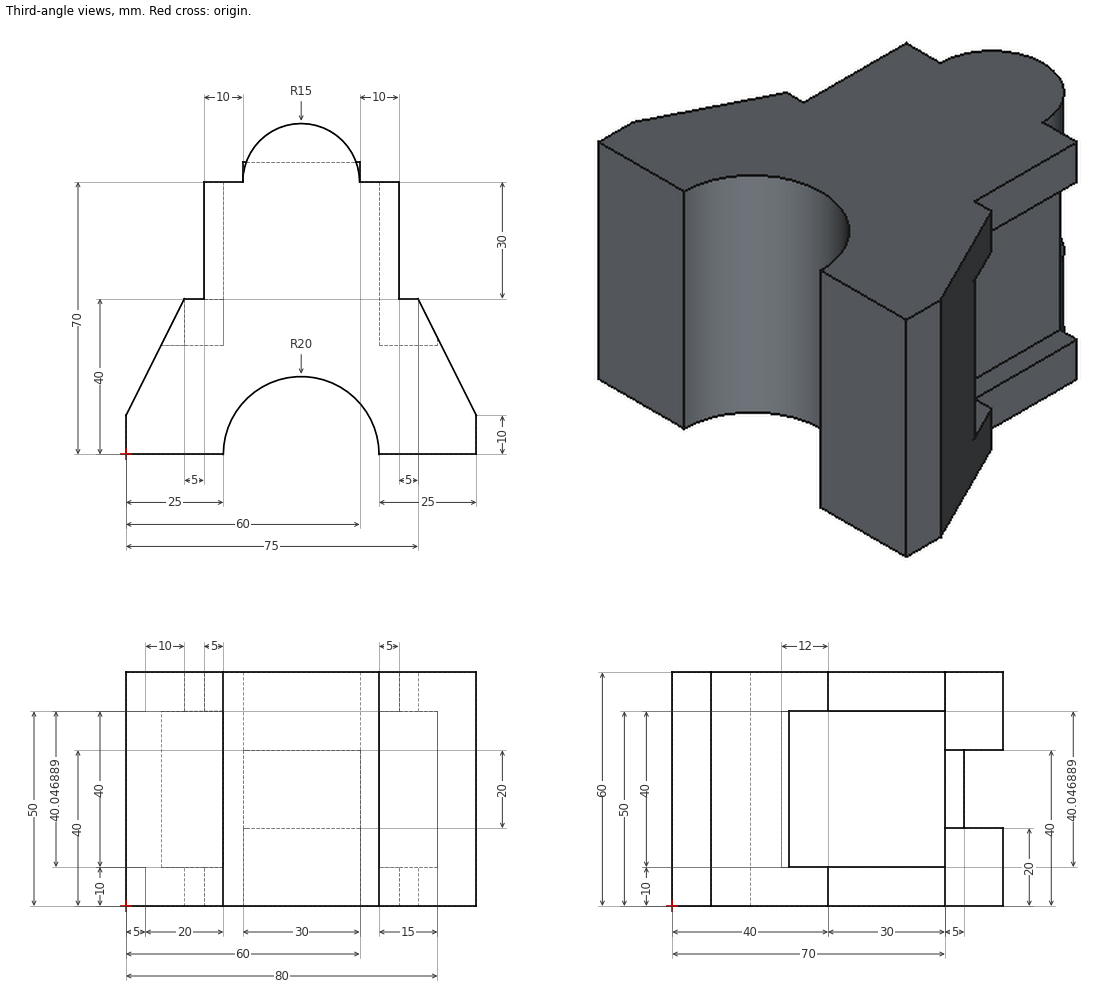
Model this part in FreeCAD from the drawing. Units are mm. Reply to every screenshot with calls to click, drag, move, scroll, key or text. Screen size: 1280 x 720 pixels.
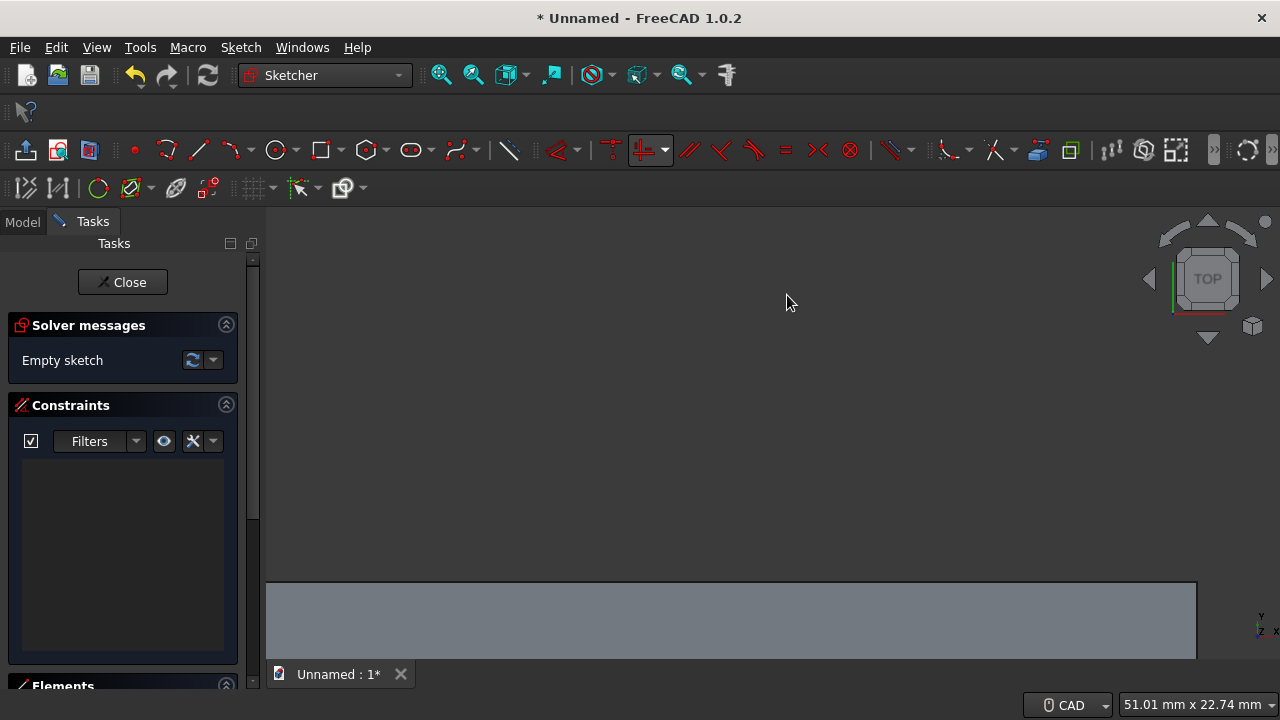
key(g)
key(l)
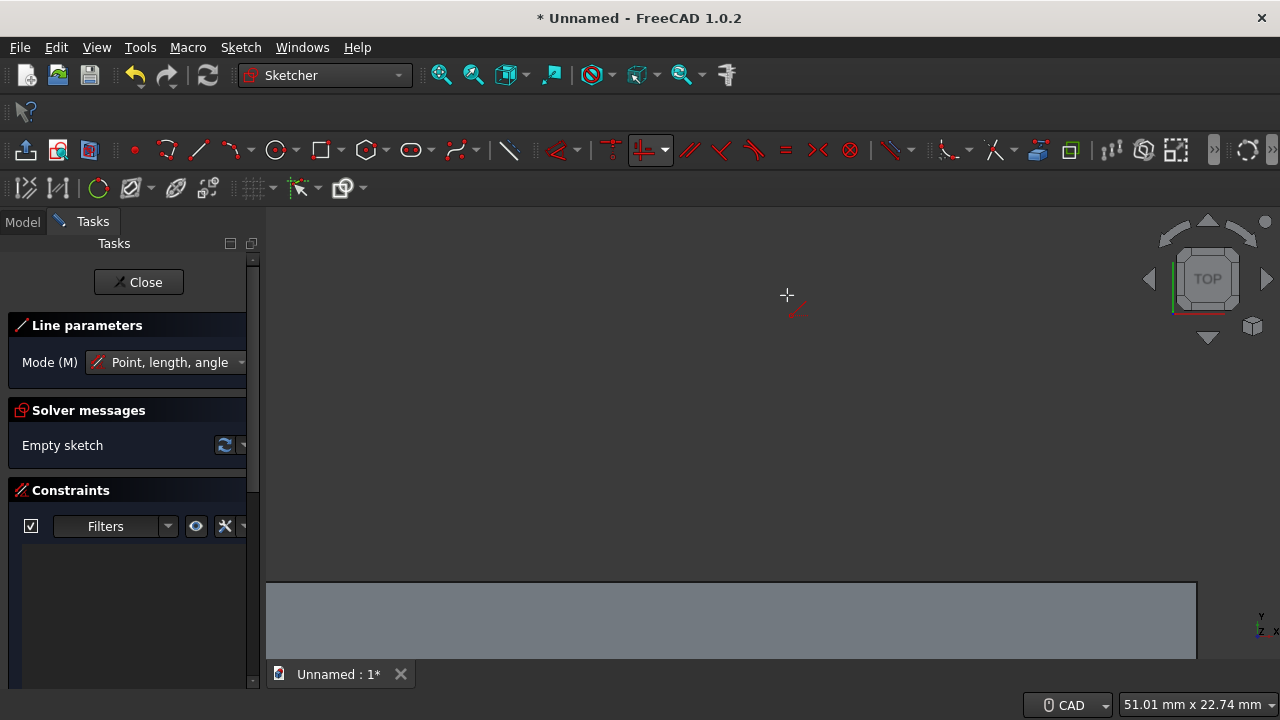
click(998, 582)
click(402, 582)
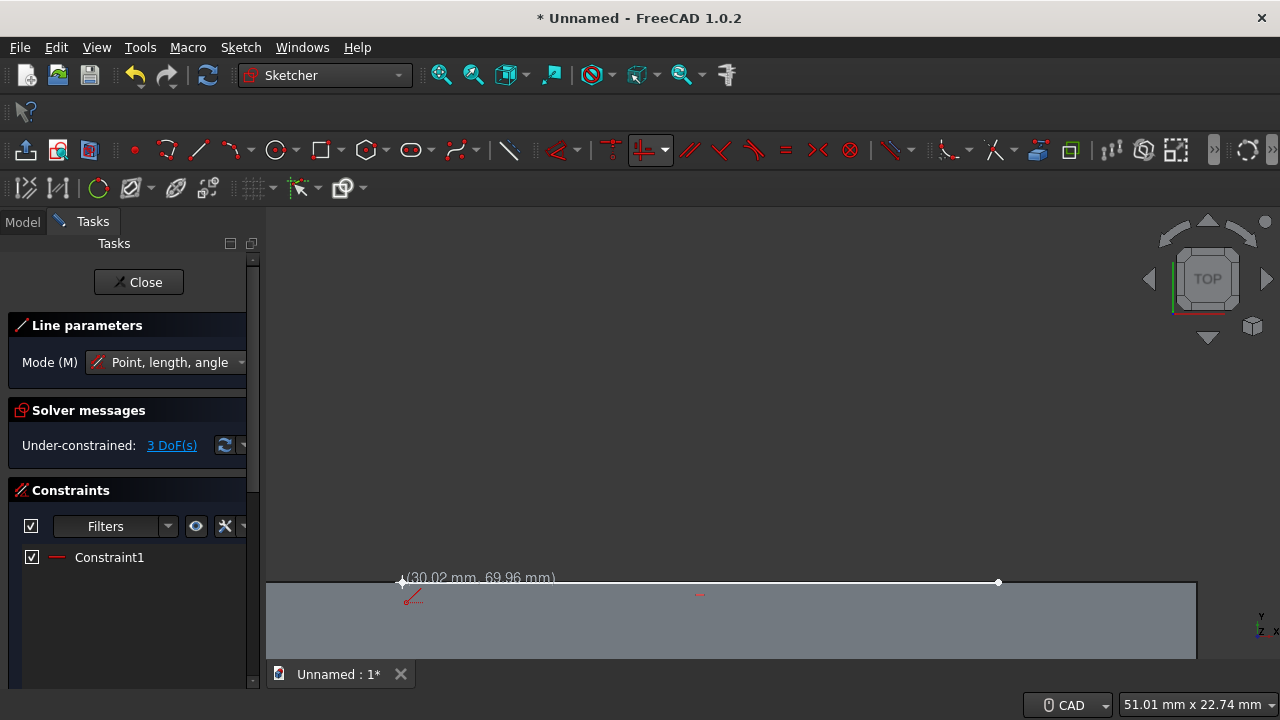
key(g)
key(3)
key(a)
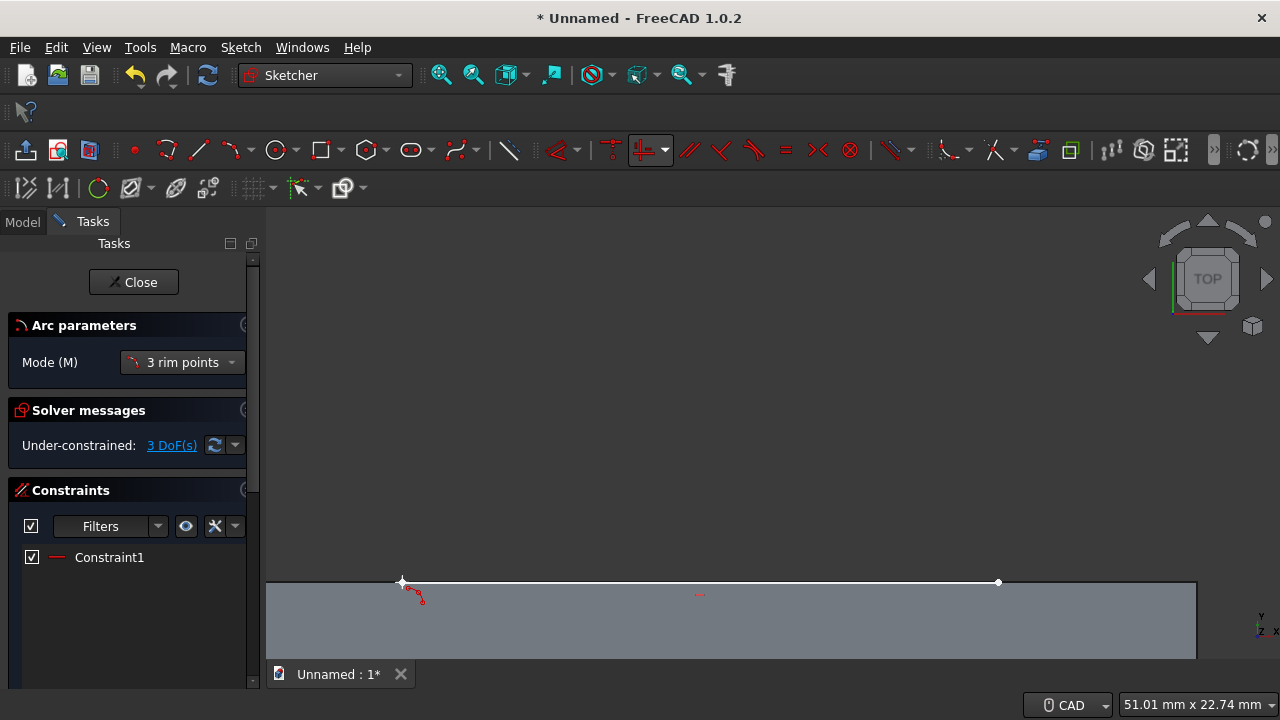
click(402, 583)
click(998, 583)
click(700, 284)
key(Escape)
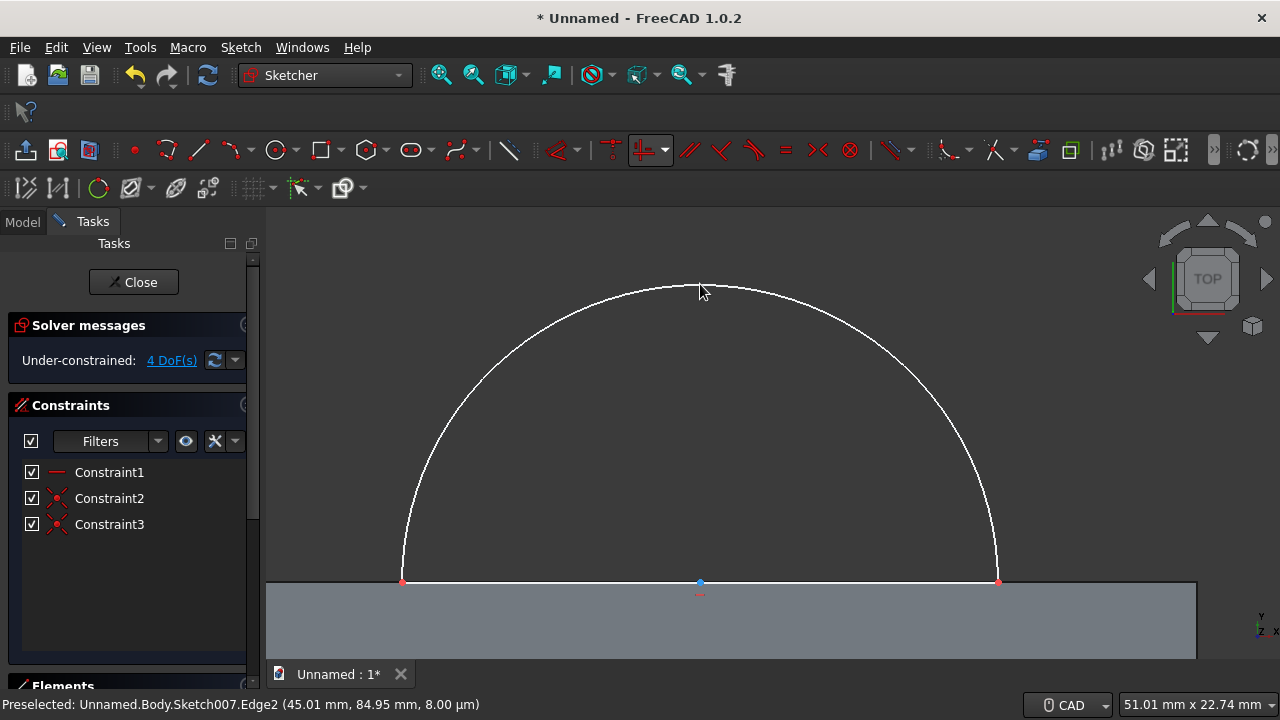
key(d)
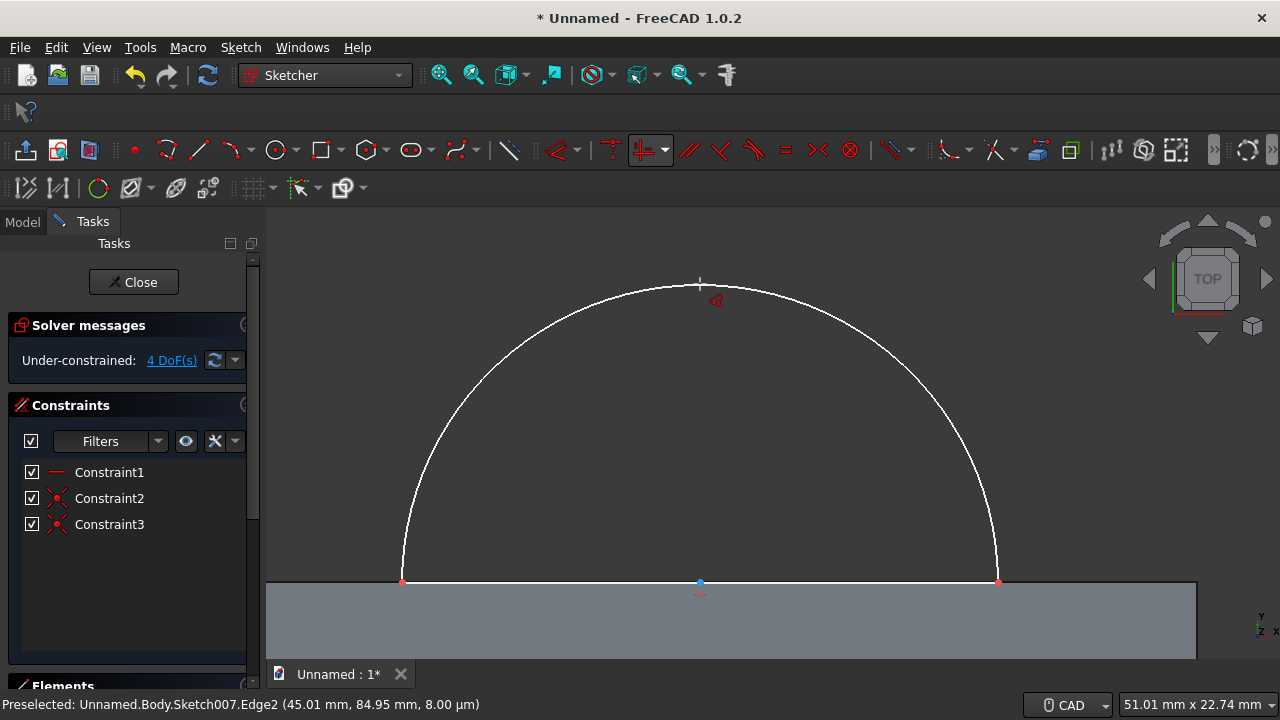
click(875, 342)
click(894, 316)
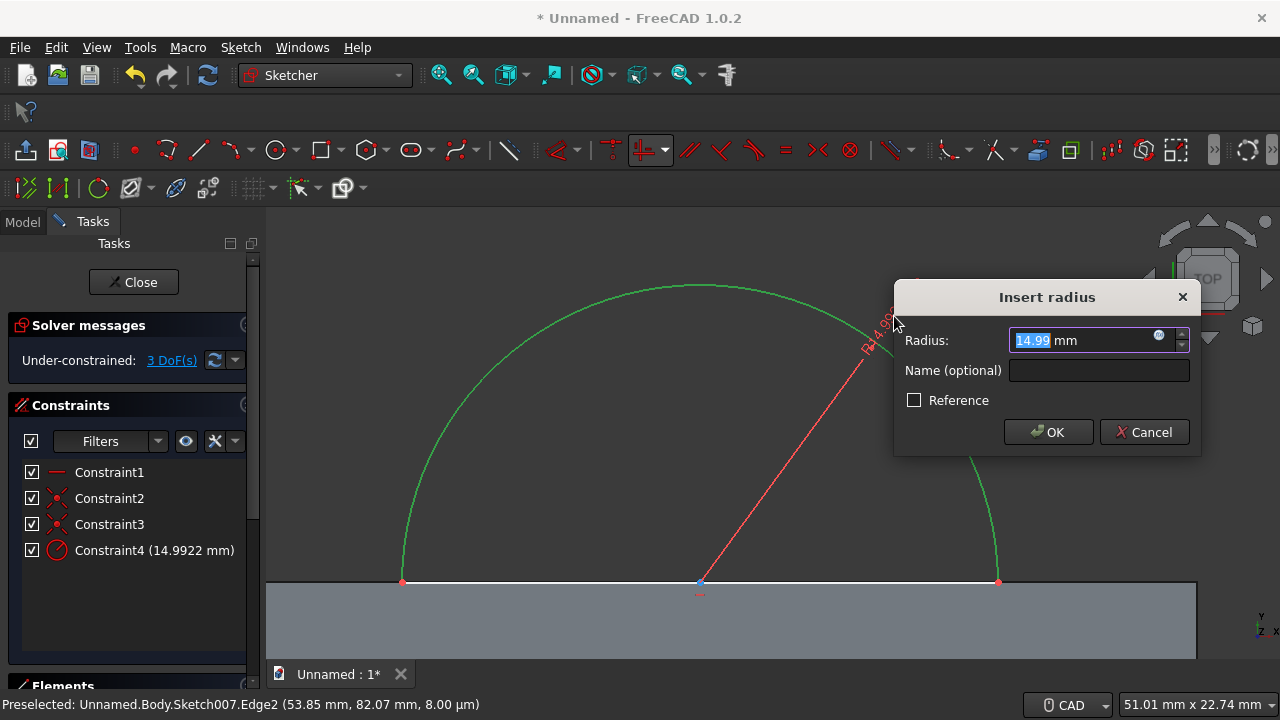
text(15)
key(Return)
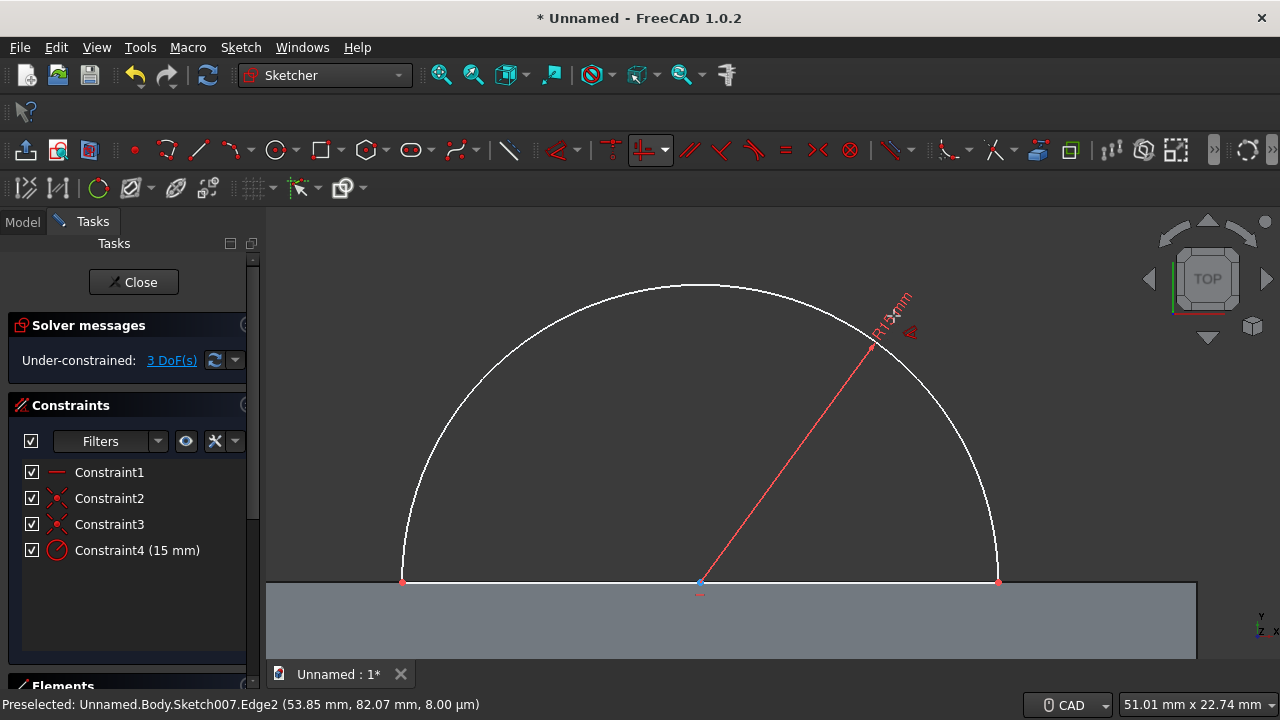
click(998, 583)
click(646, 549)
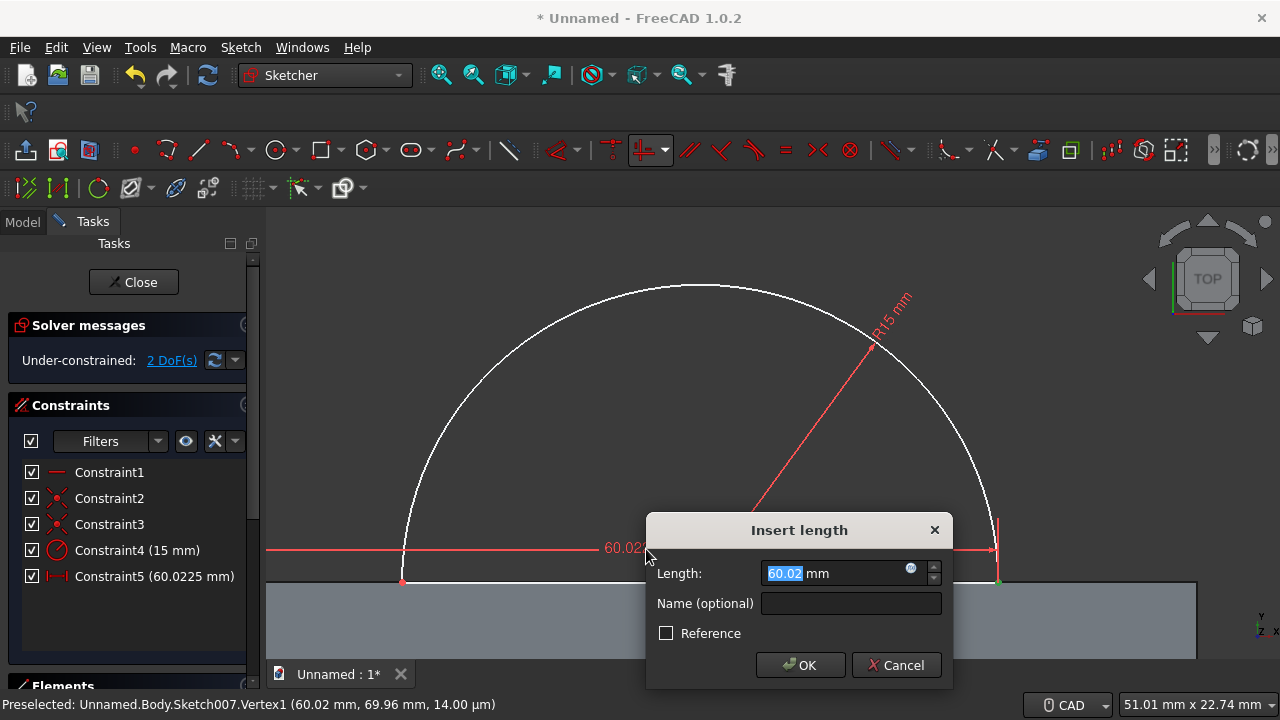
text(60)
key(Return)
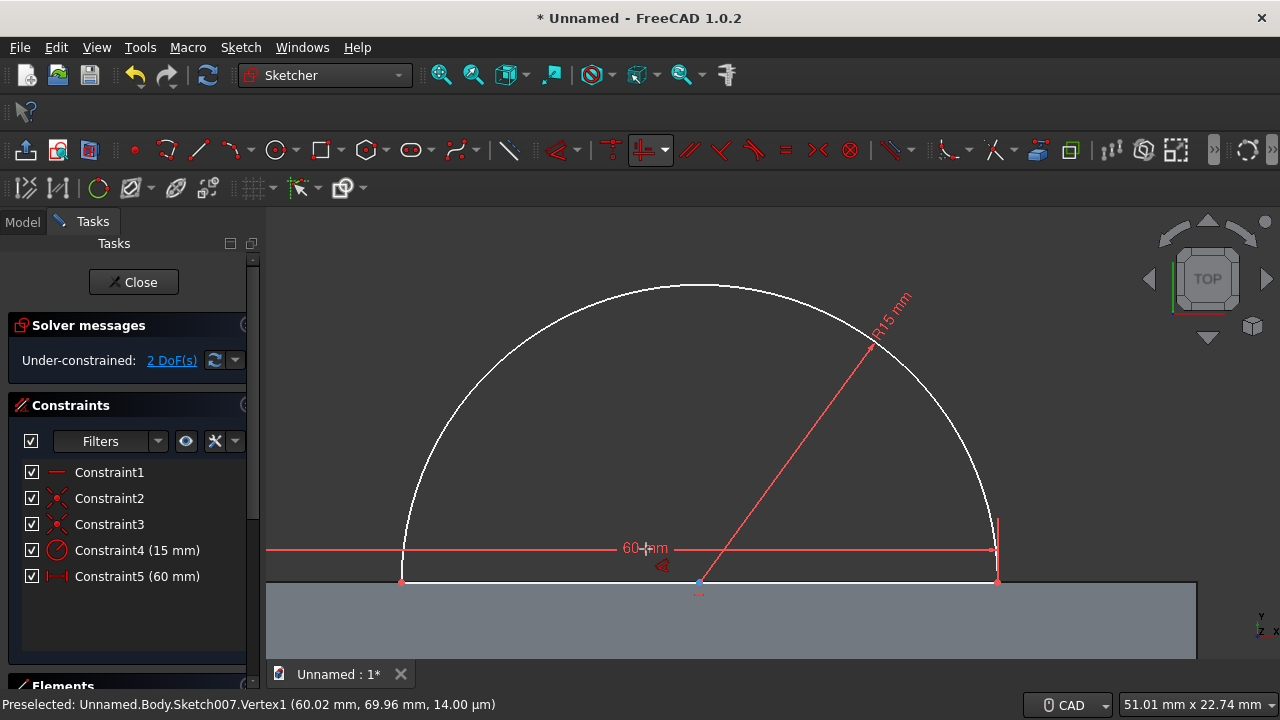
click(998, 583)
click(1032, 607)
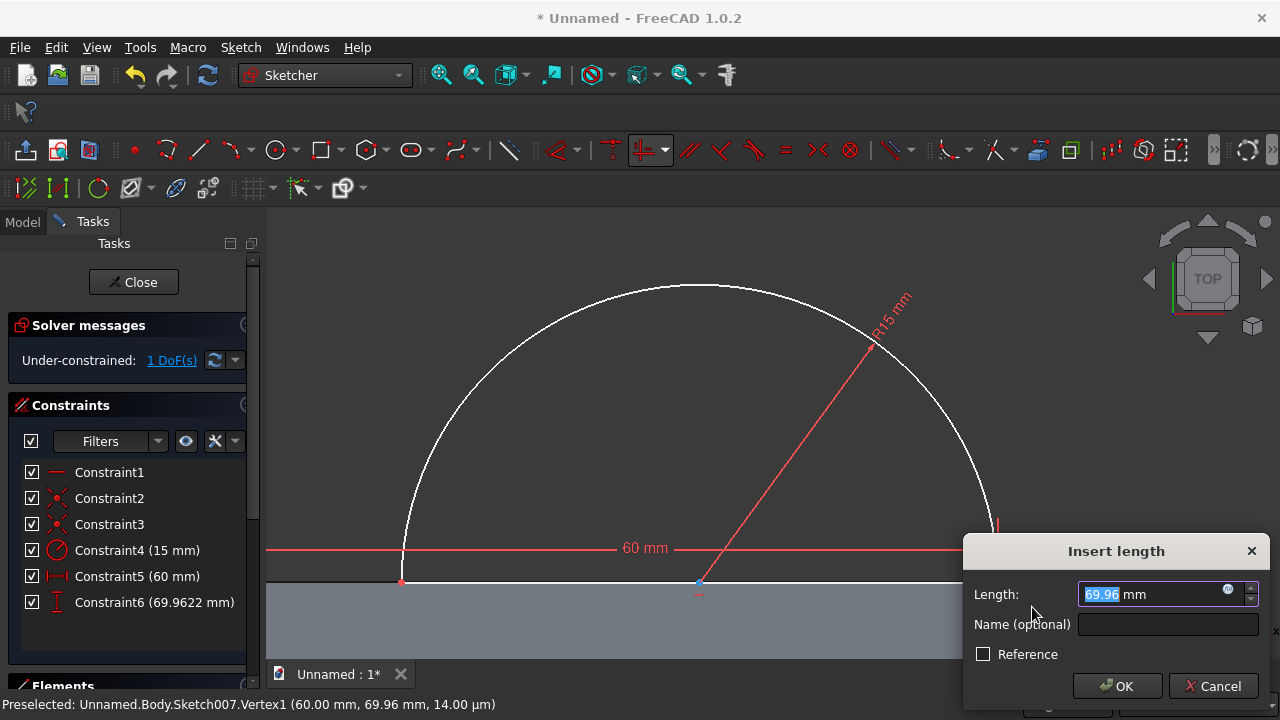
text(70)
key(Return)